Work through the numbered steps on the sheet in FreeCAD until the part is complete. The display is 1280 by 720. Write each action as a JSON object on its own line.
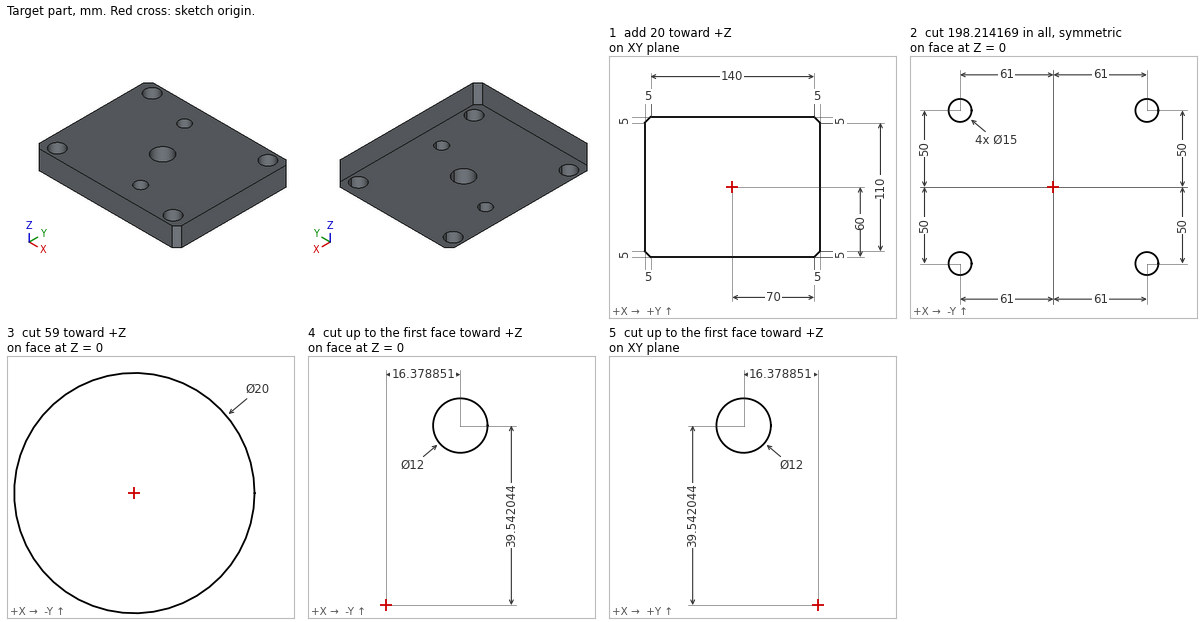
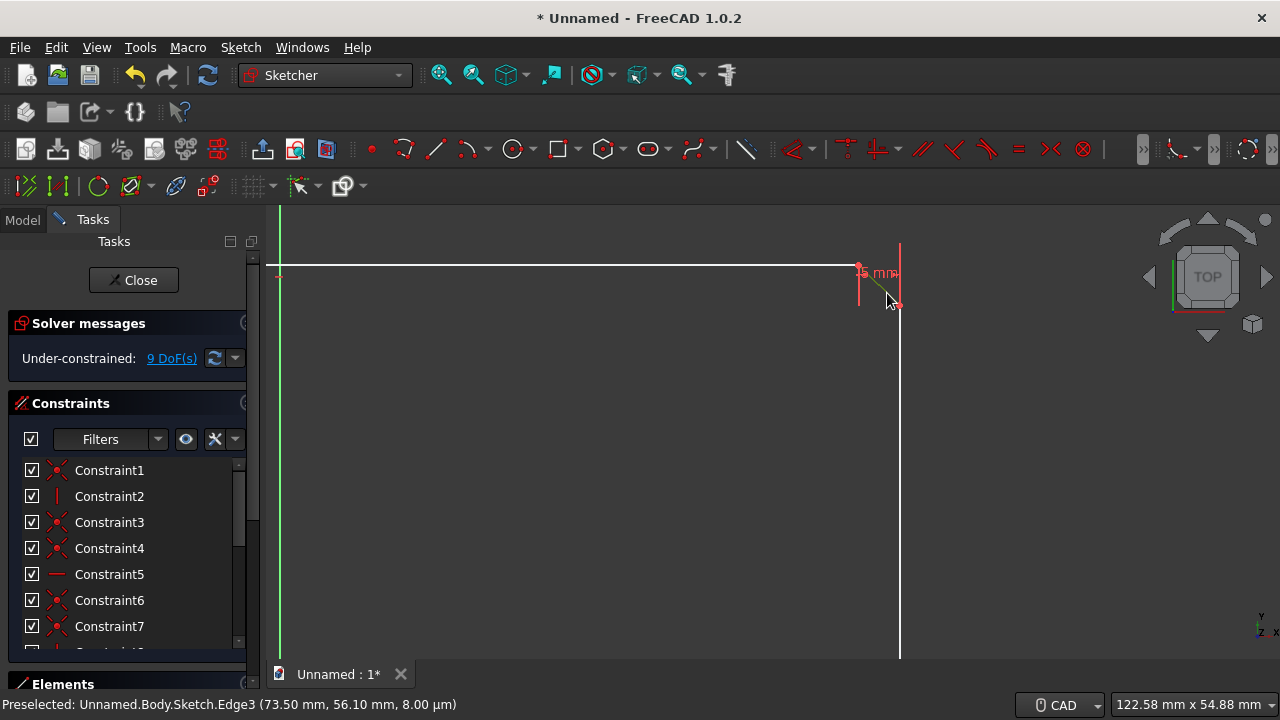
{"action": "left_click", "coordinate": [814, 150]}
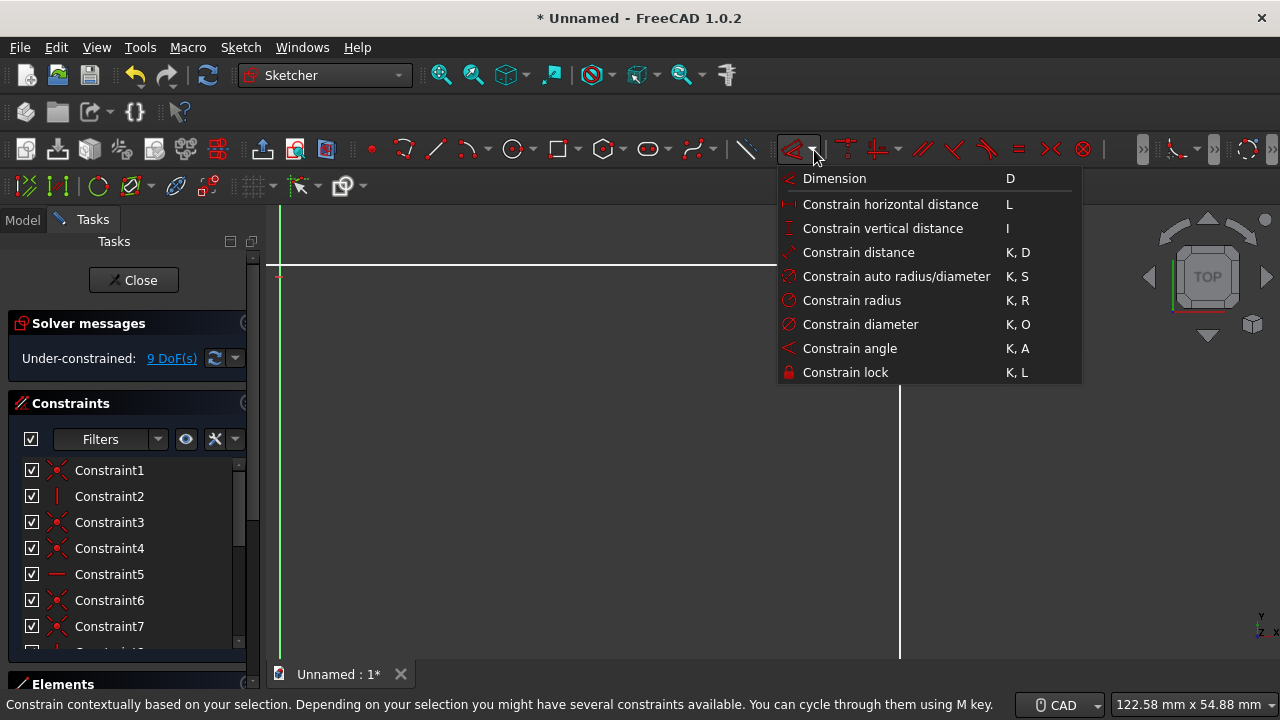
{"action": "left_click", "coordinate": [930, 228]}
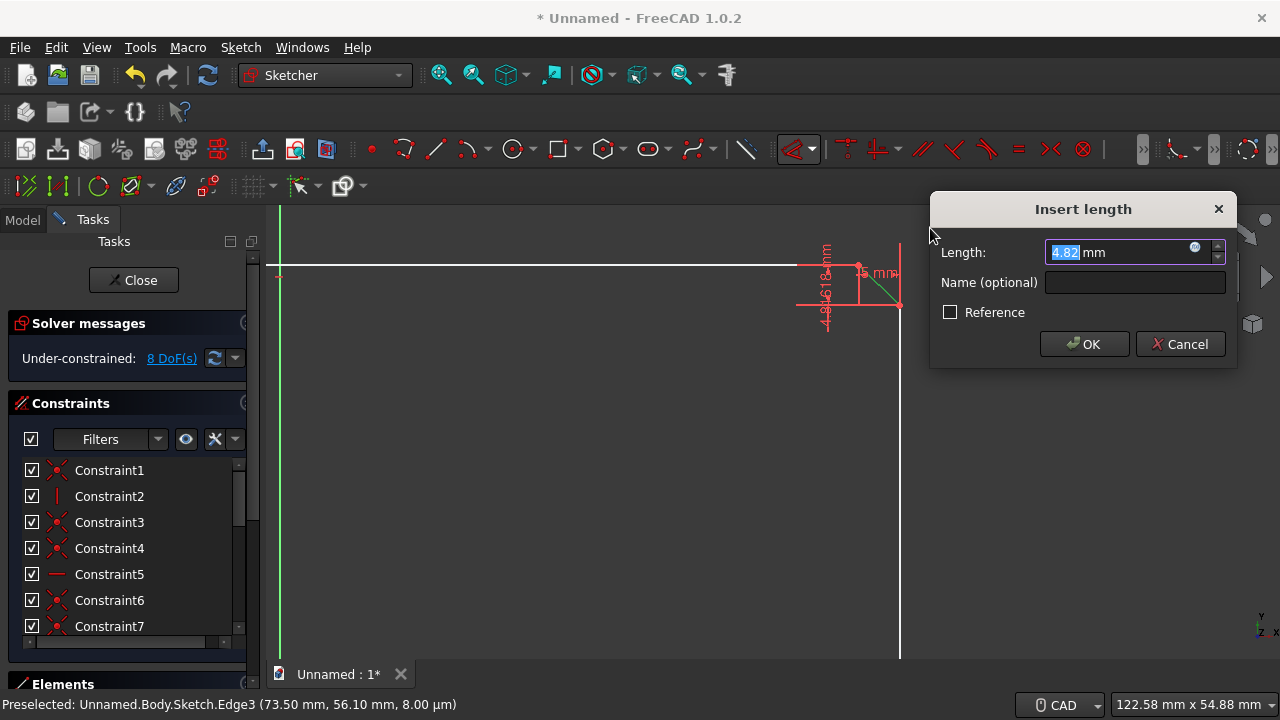
{"action": "type", "text": "5"}
{"action": "key", "text": "Return"}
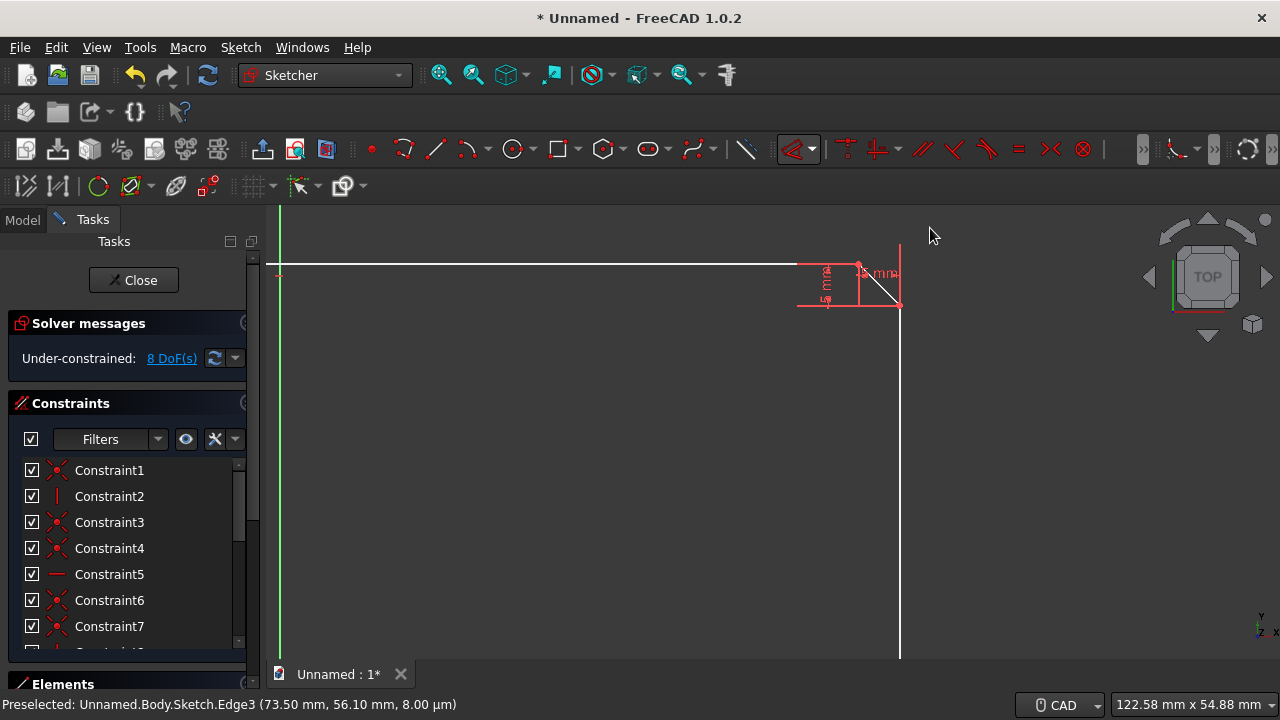
{"action": "scroll", "coordinate": [888, 292], "scroll_direction": "down", "scroll_amount": 6}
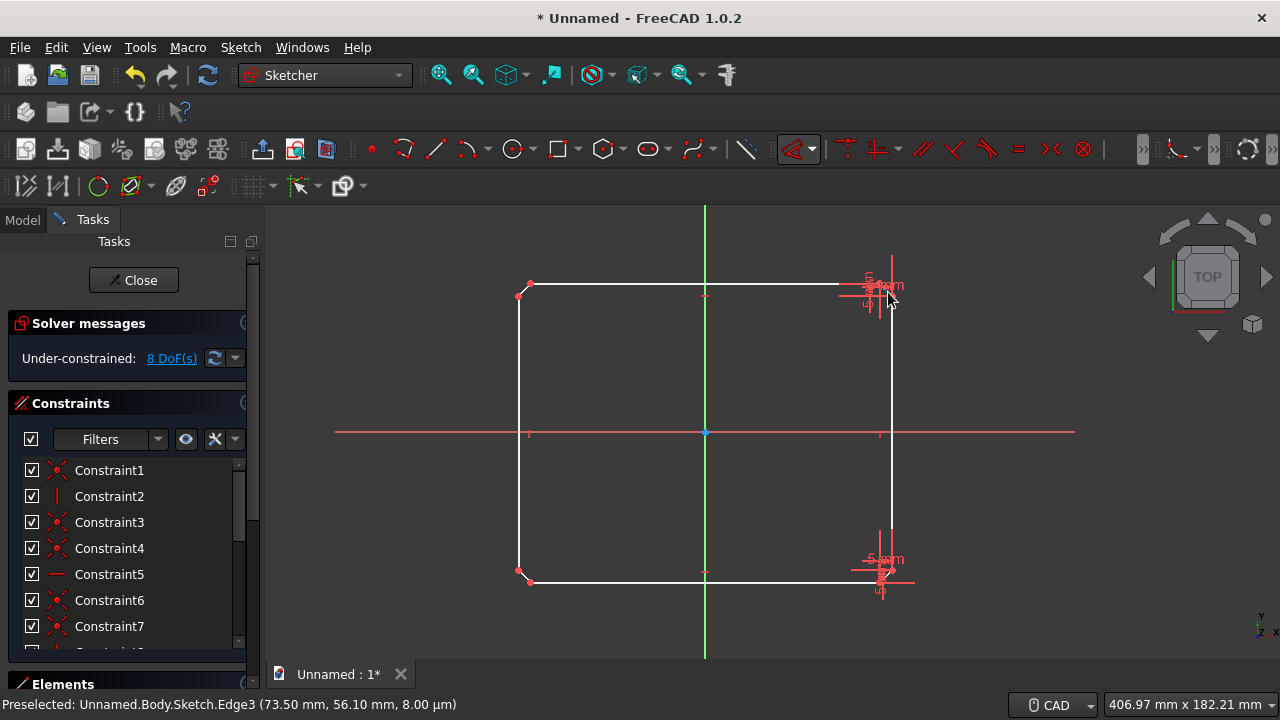
{"action": "scroll", "coordinate": [527, 287], "scroll_direction": "up", "scroll_amount": 6}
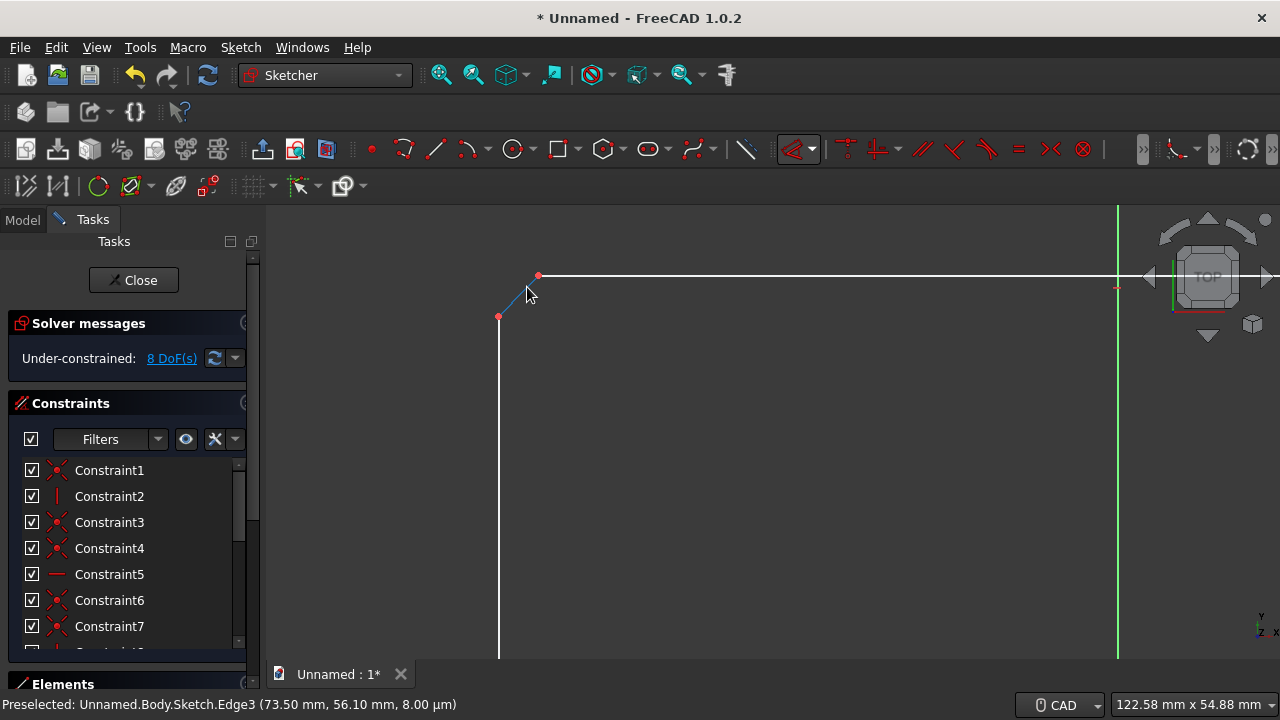
{"action": "left_click", "coordinate": [526, 288]}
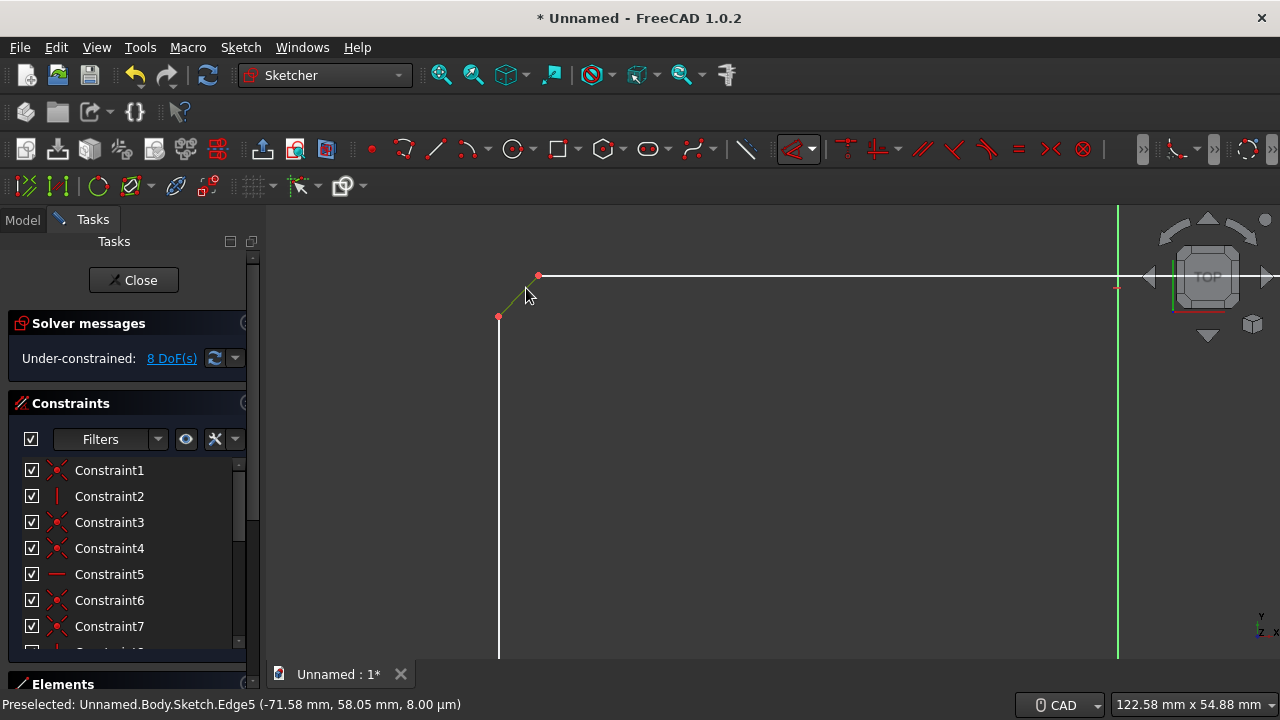
{"action": "key", "text": "l"}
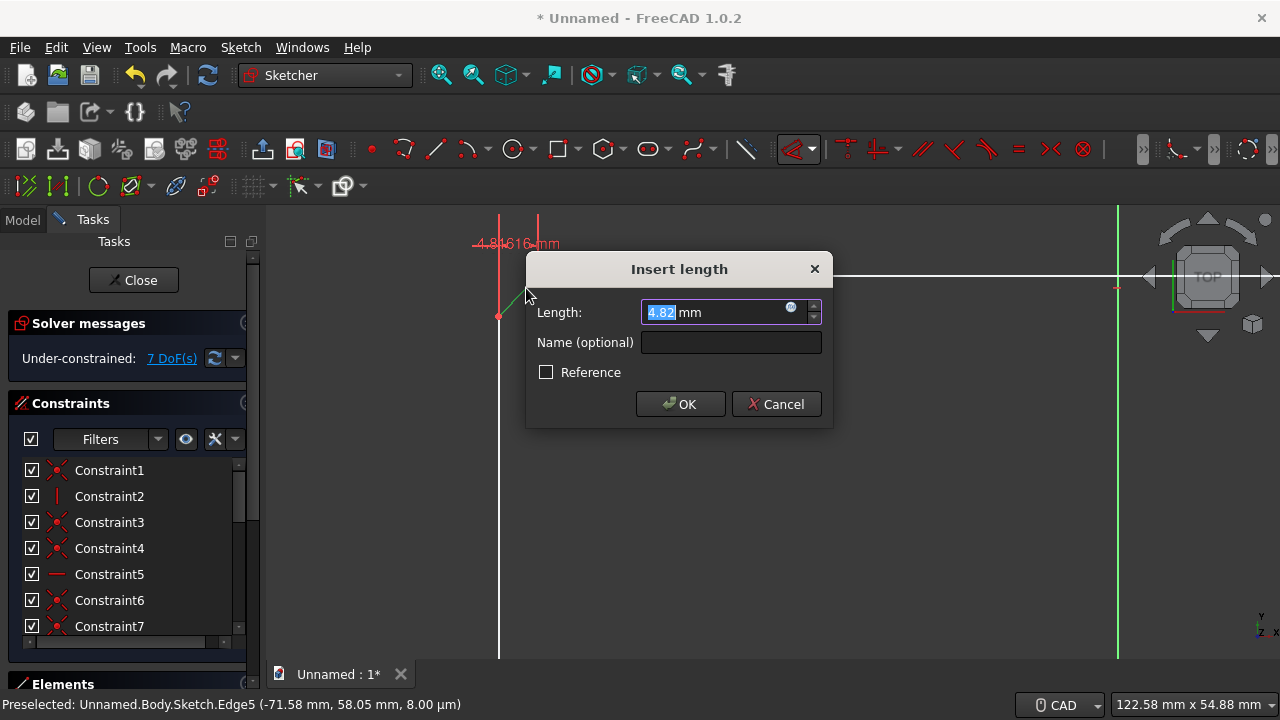
{"action": "type", "text": "5"}
{"action": "key", "text": "Return"}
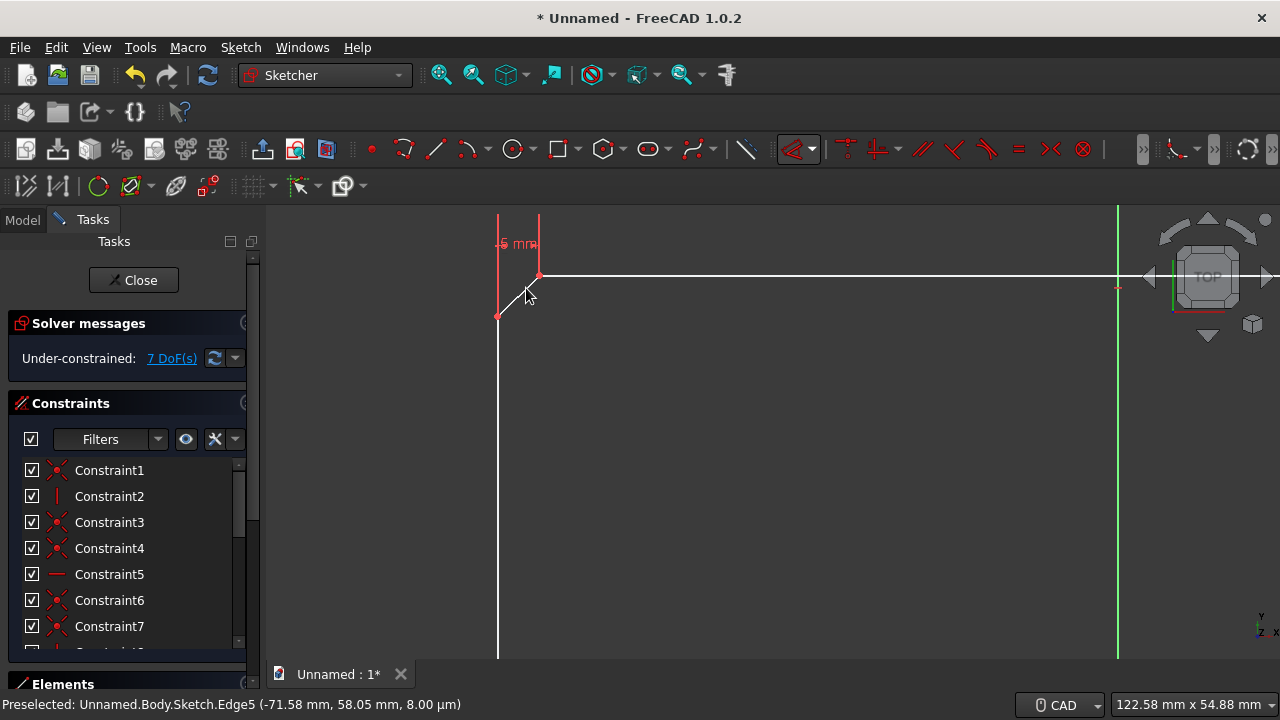
{"action": "left_click", "coordinate": [527, 288]}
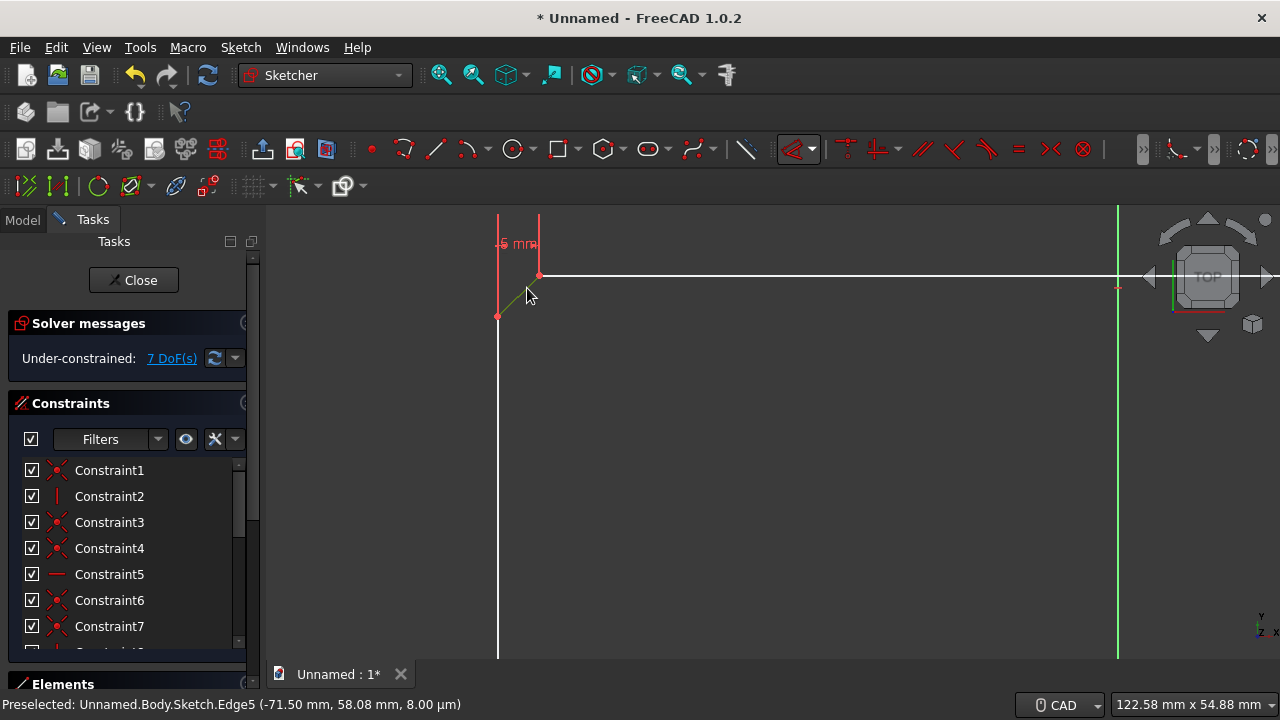
{"action": "left_click", "coordinate": [814, 150]}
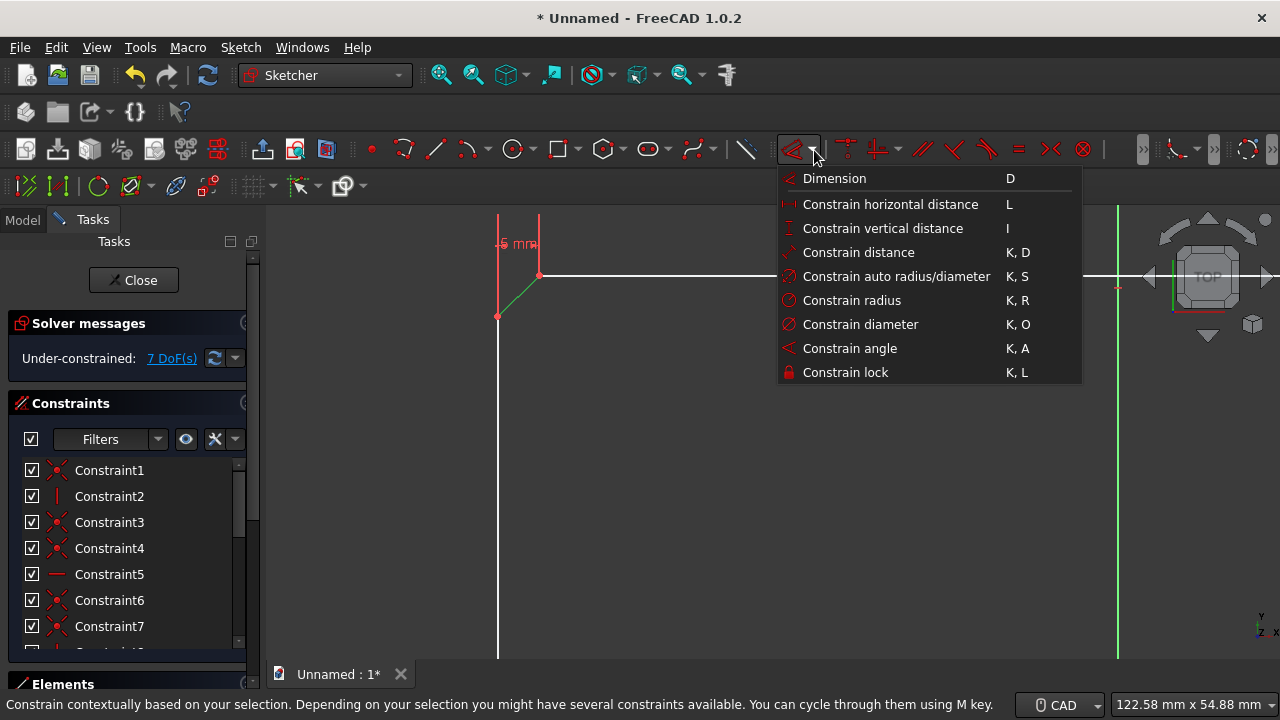
{"action": "left_click", "coordinate": [930, 228]}